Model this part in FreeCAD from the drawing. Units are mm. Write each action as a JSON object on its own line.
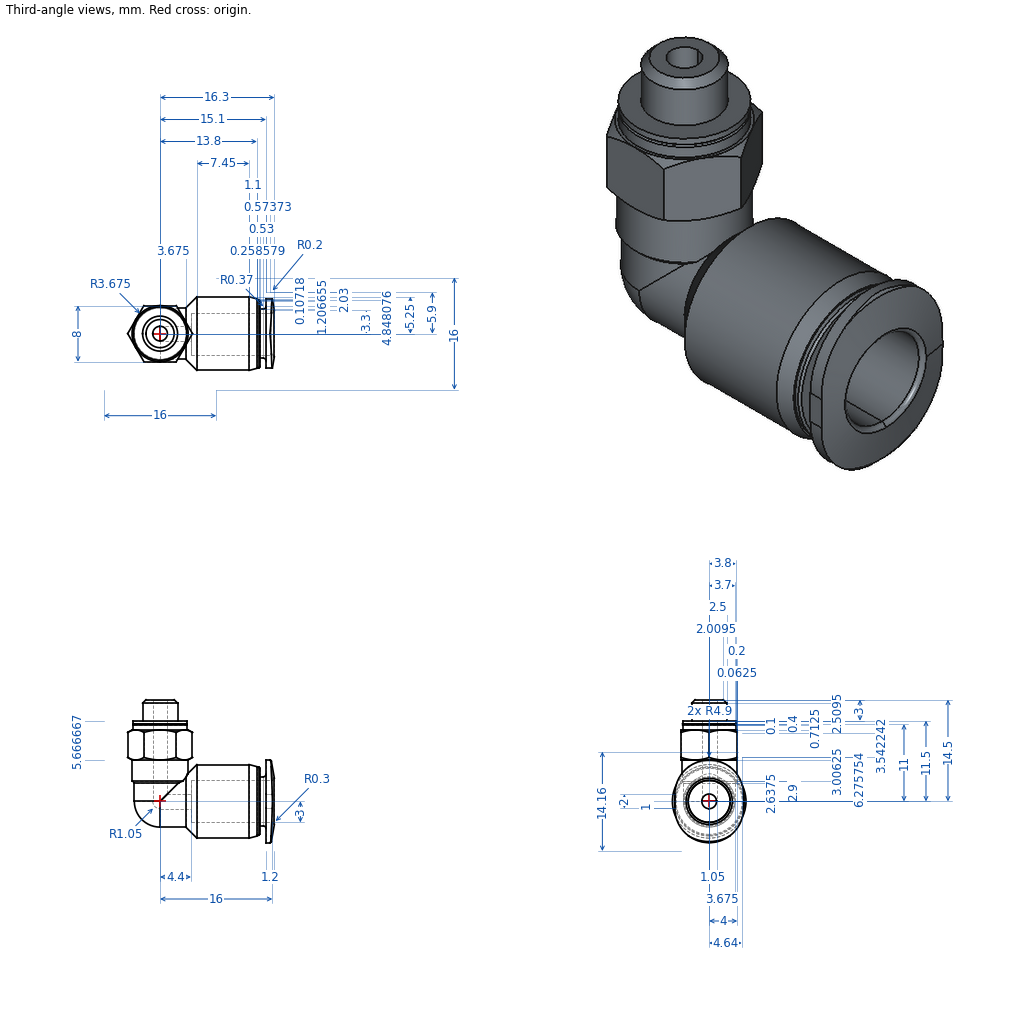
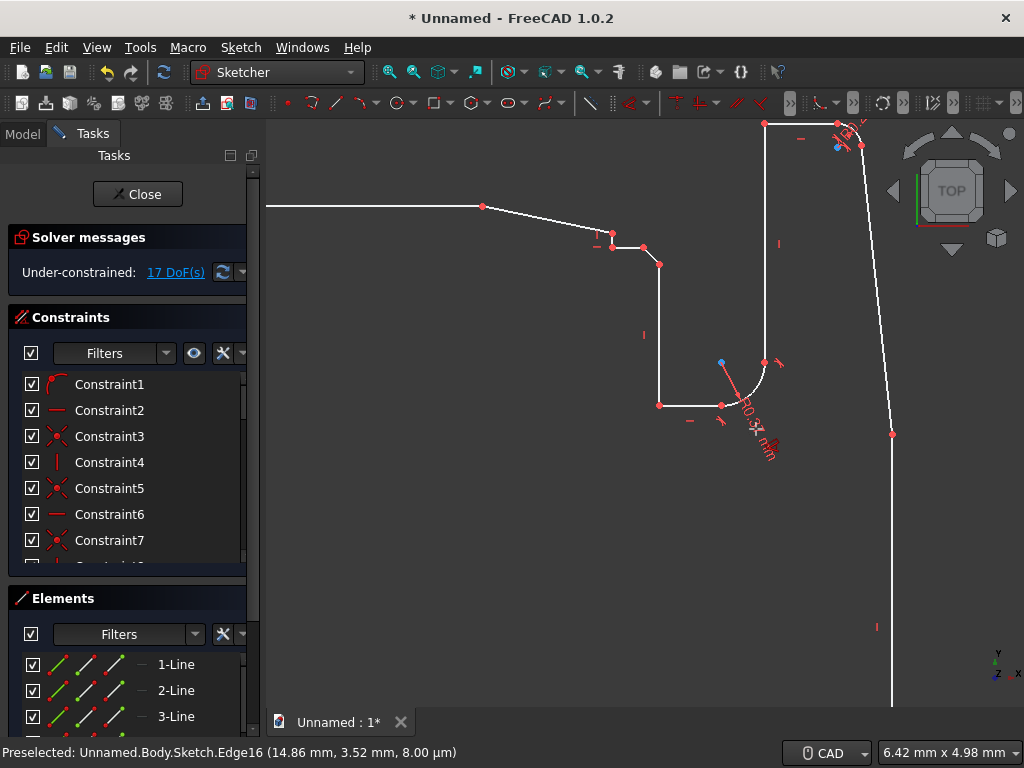
{"action": "scroll", "coordinate": [745, 402], "scroll_direction": "down", "scroll_amount": 9}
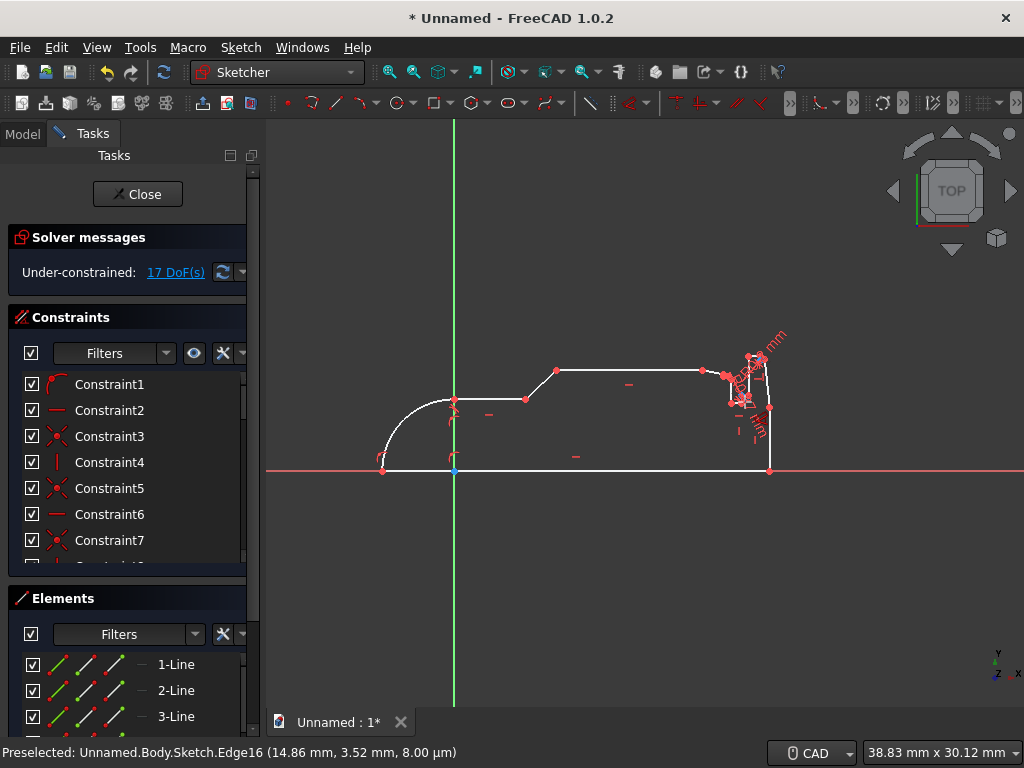
{"action": "left_click", "coordinate": [422, 407]}
{"action": "left_click", "coordinate": [408, 378]}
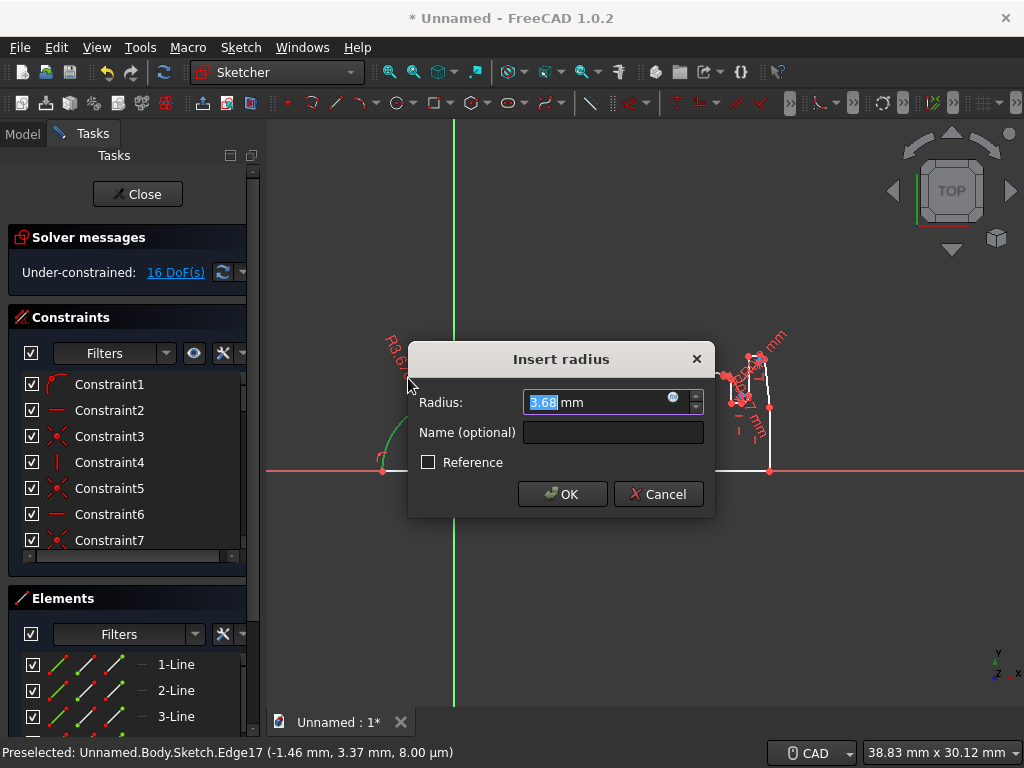
{"action": "type", "text": "3.675"}
{"action": "key", "text": "Return"}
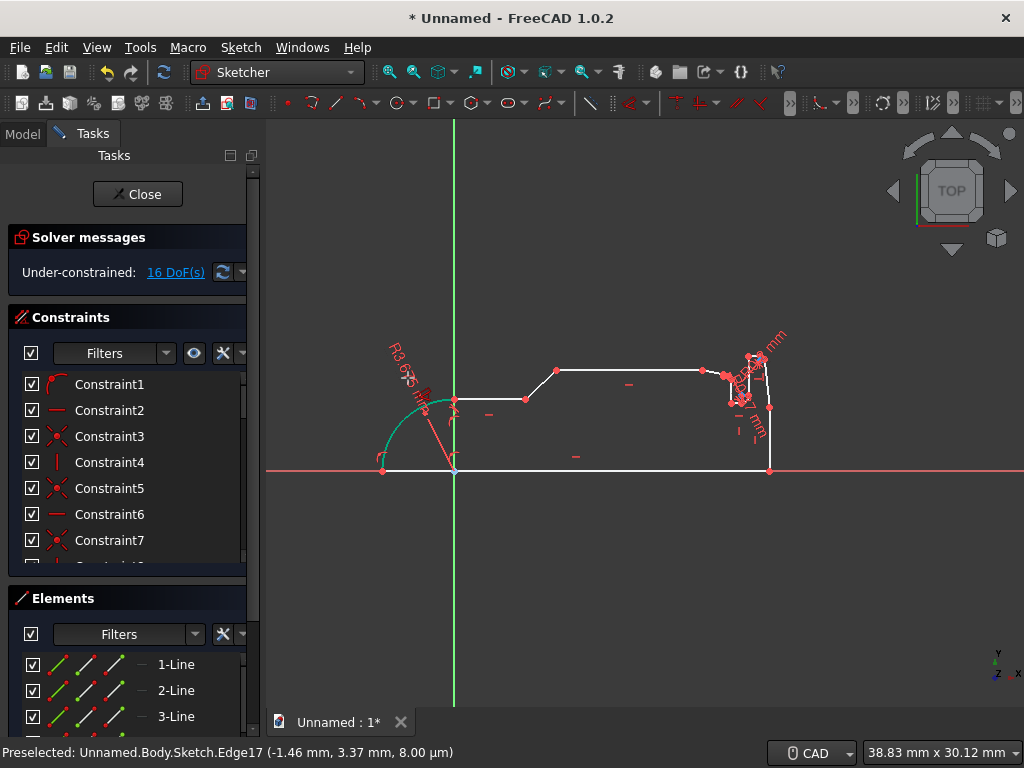
{"action": "left_click", "coordinate": [770, 452]}
{"action": "left_click", "coordinate": [804, 439]}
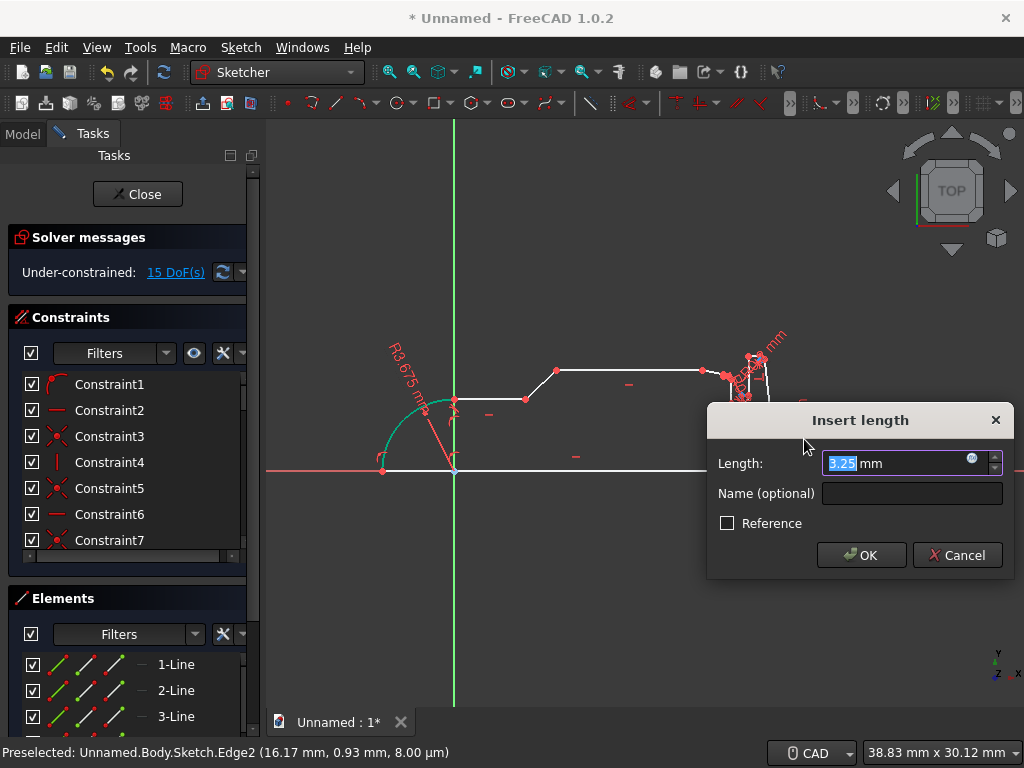
{"action": "type", "text": "3.3"}
{"action": "key", "text": "Return"}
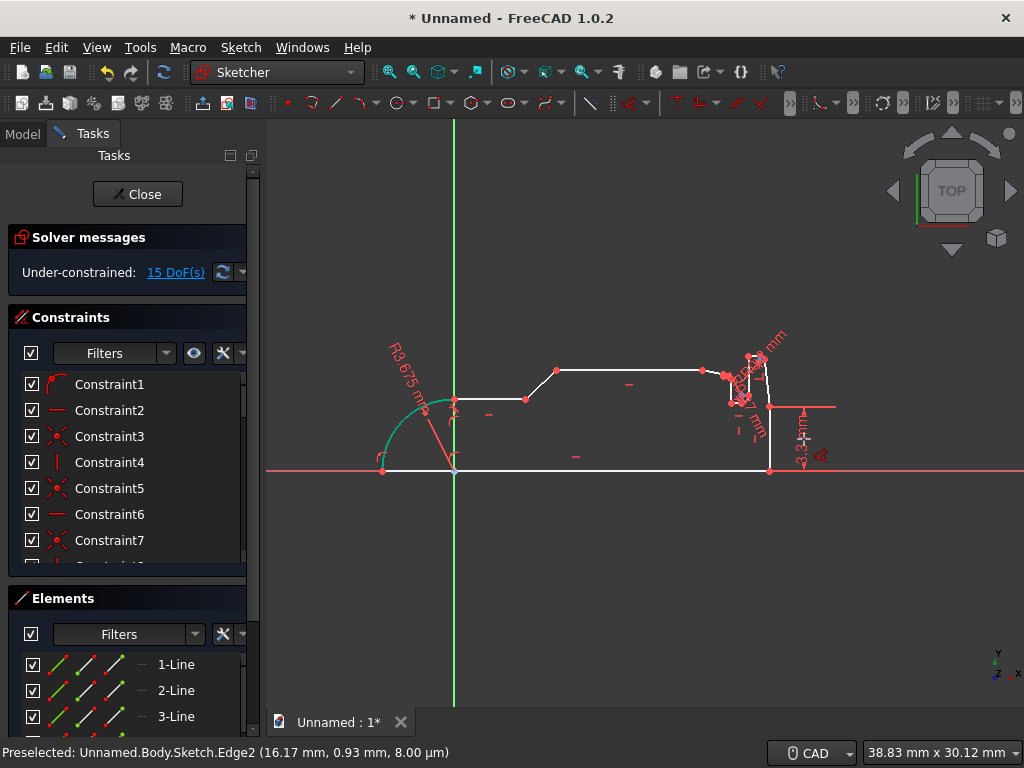
{"action": "left_click", "coordinate": [749, 368]}
{"action": "left_click", "coordinate": [783, 376]}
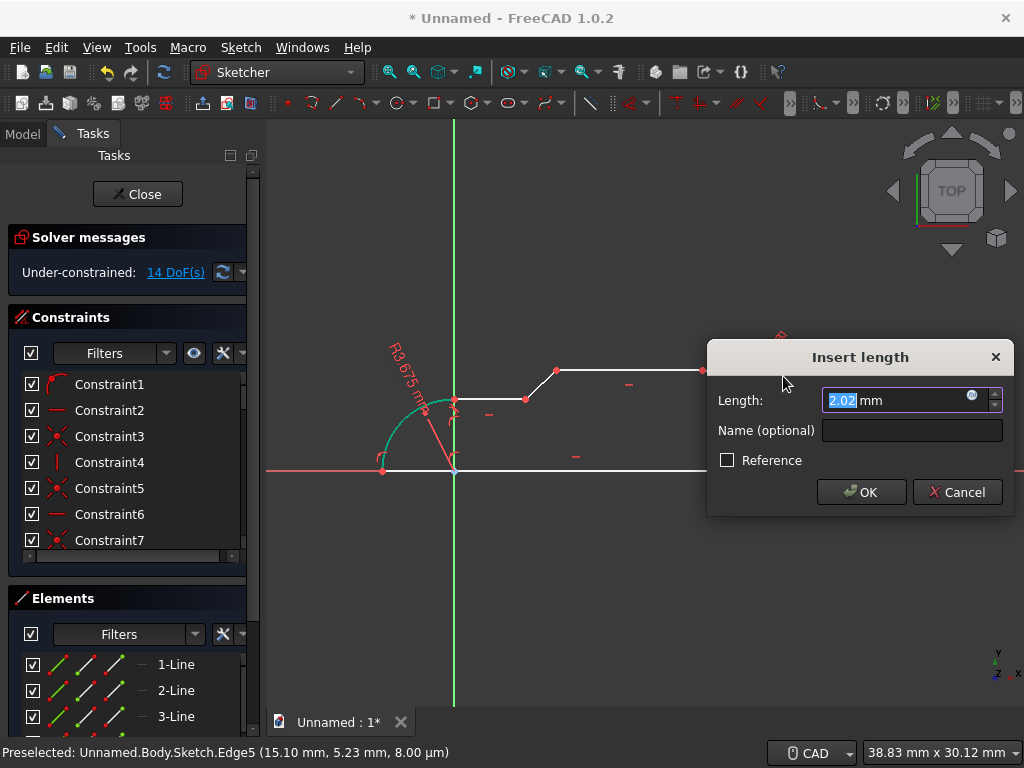
{"action": "type", "text": "2.03"}
{"action": "key", "text": "Return"}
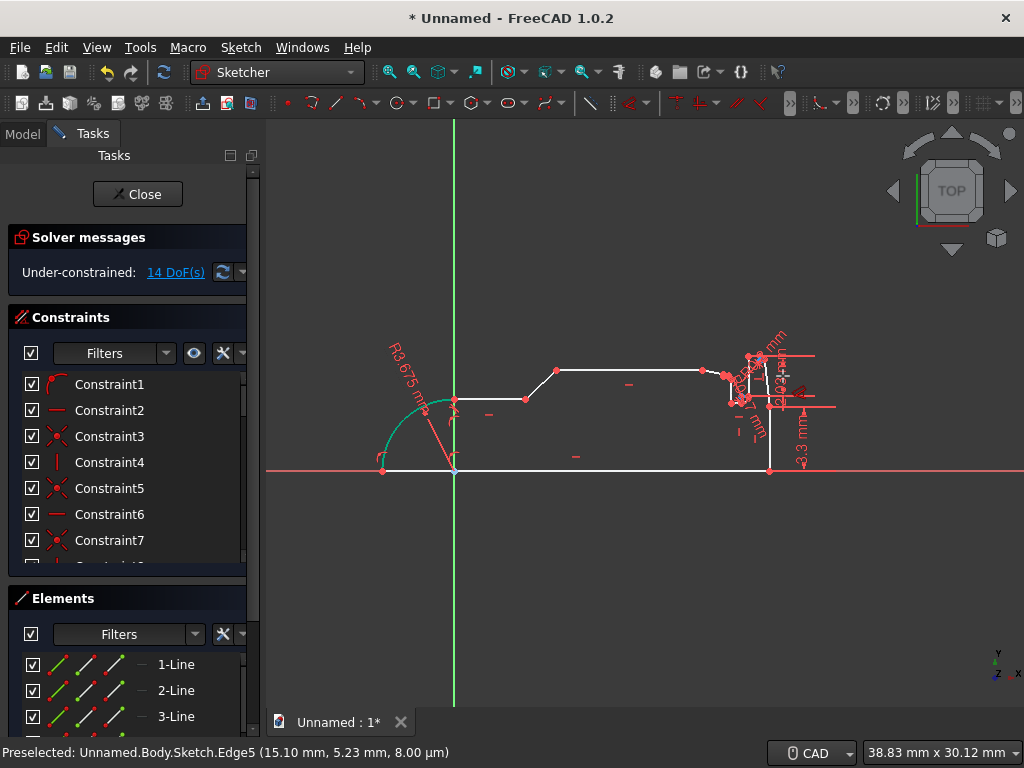
{"action": "scroll", "coordinate": [736, 403], "scroll_direction": "up", "scroll_amount": 7}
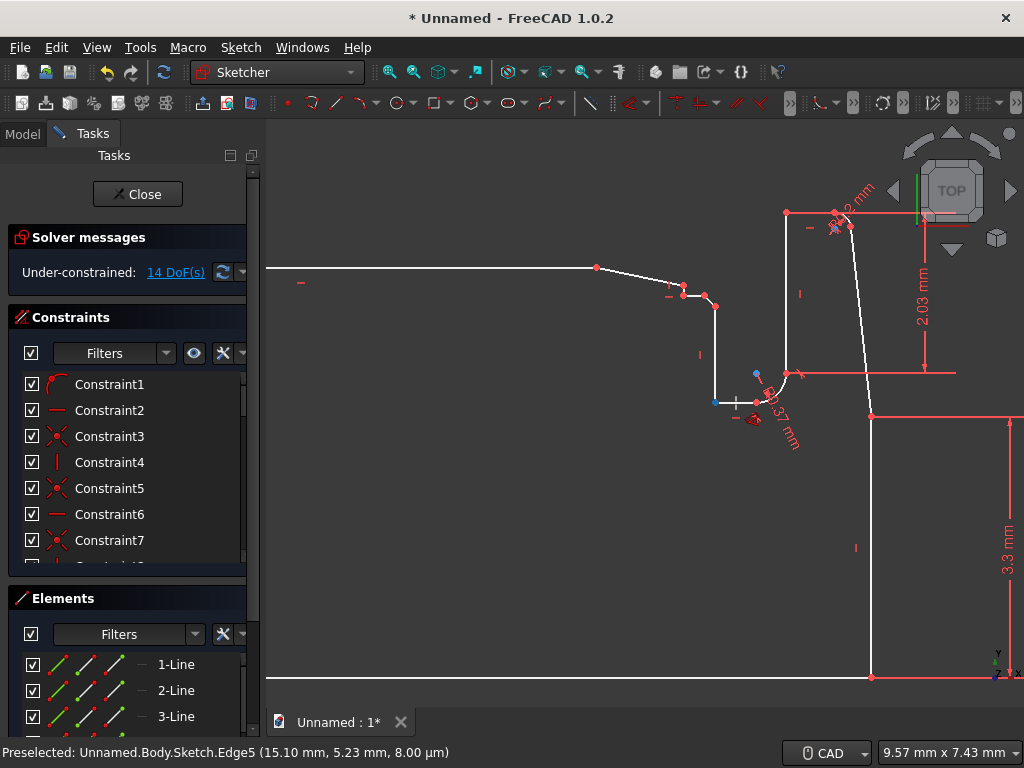
{"action": "left_click", "coordinate": [736, 403]}
{"action": "left_click", "coordinate": [736, 369]}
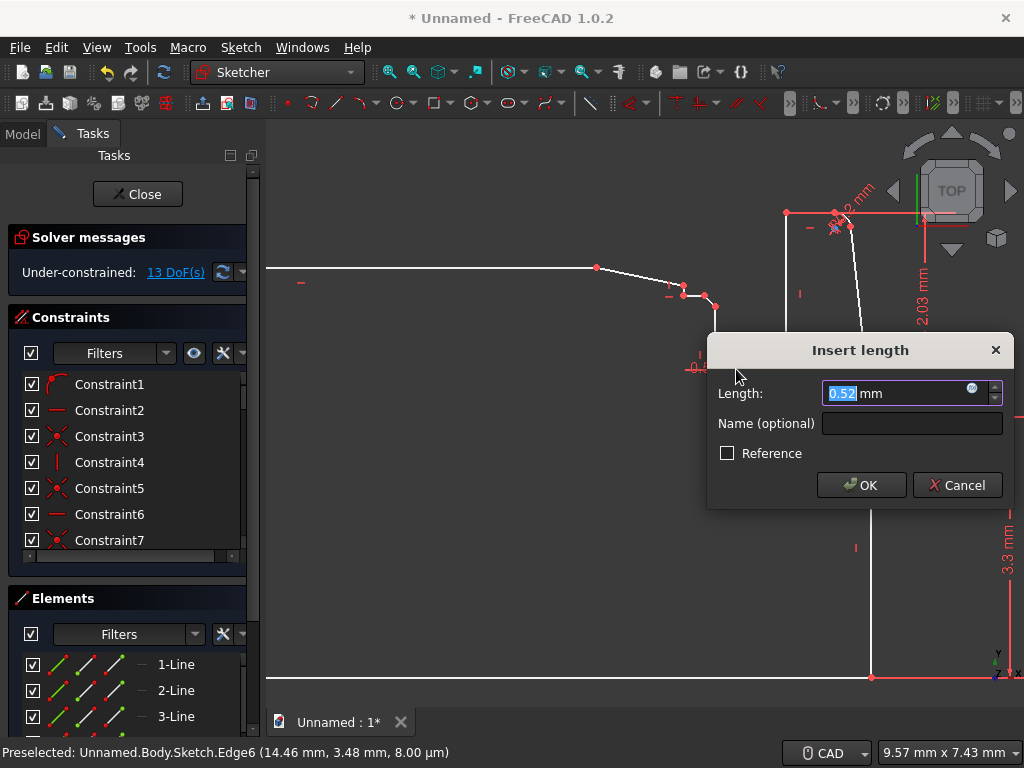
{"action": "type", "text": "0.53"}
{"action": "key", "text": "Return"}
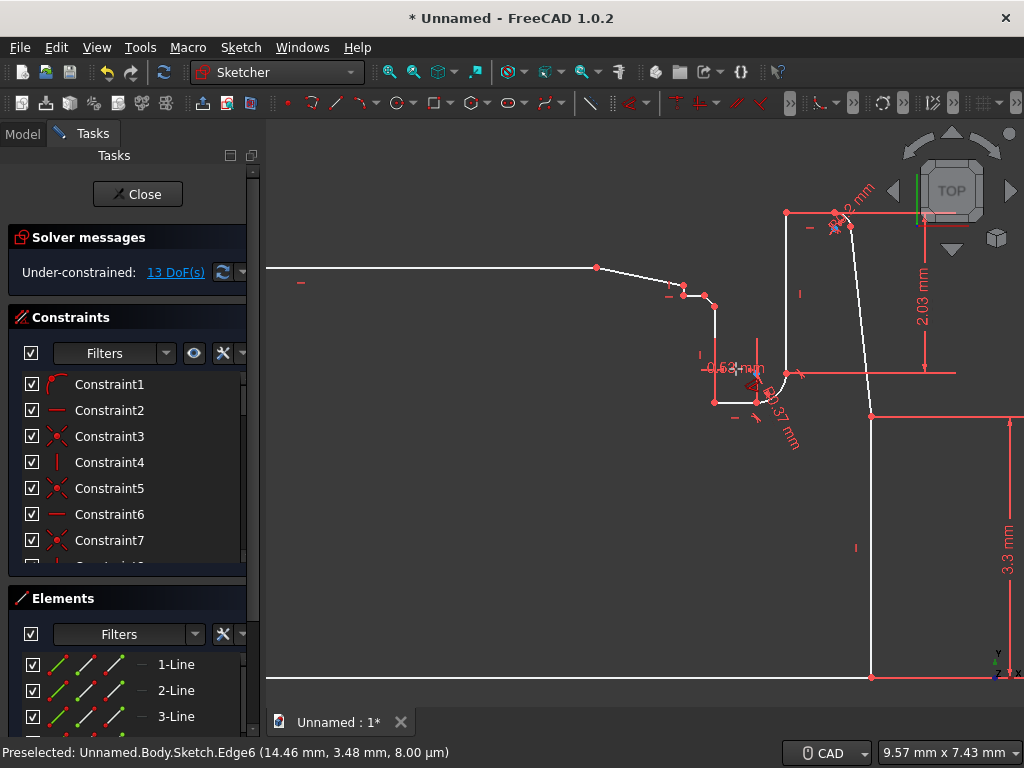
{"action": "scroll", "coordinate": [736, 403], "scroll_direction": "down", "scroll_amount": 7}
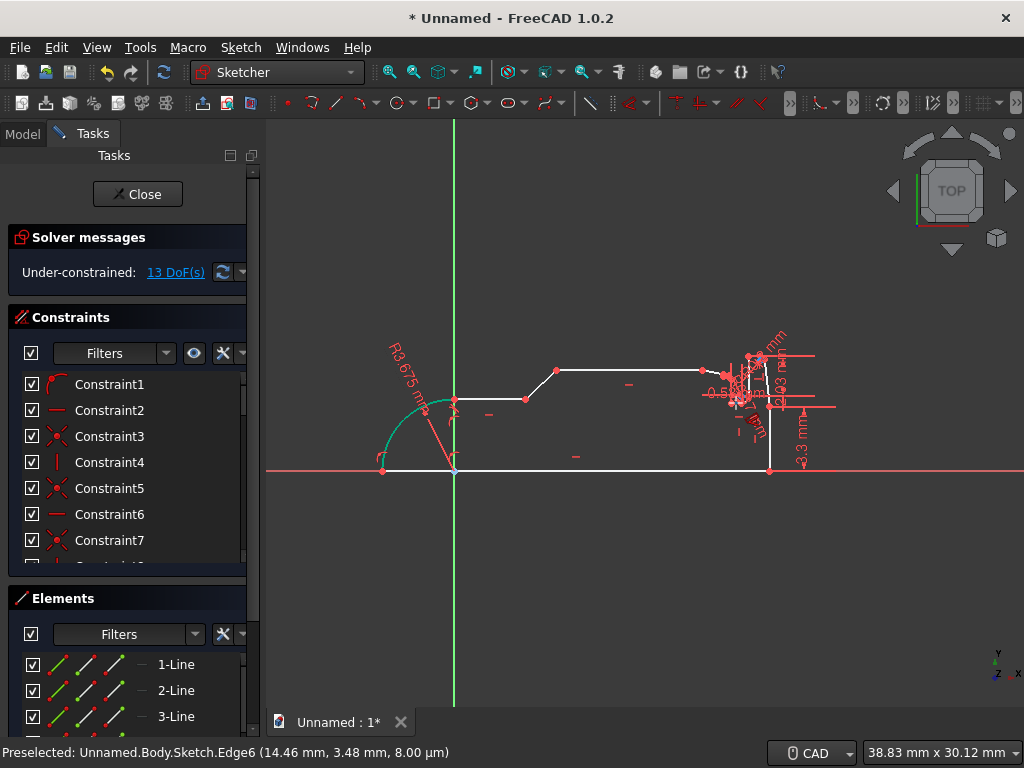
{"action": "left_click", "coordinate": [659, 370]}
{"action": "left_click", "coordinate": [629, 336]}